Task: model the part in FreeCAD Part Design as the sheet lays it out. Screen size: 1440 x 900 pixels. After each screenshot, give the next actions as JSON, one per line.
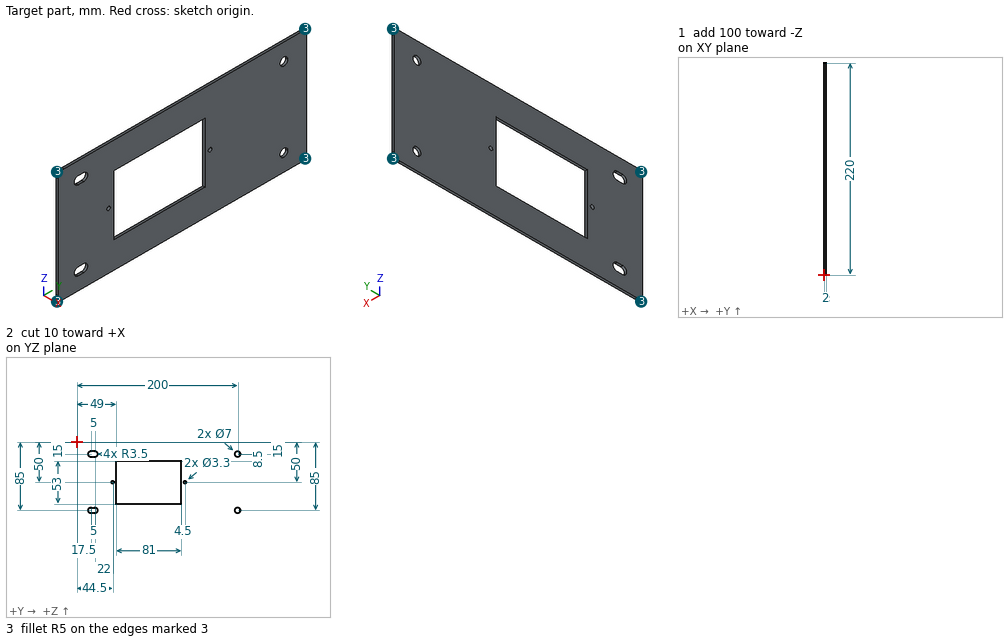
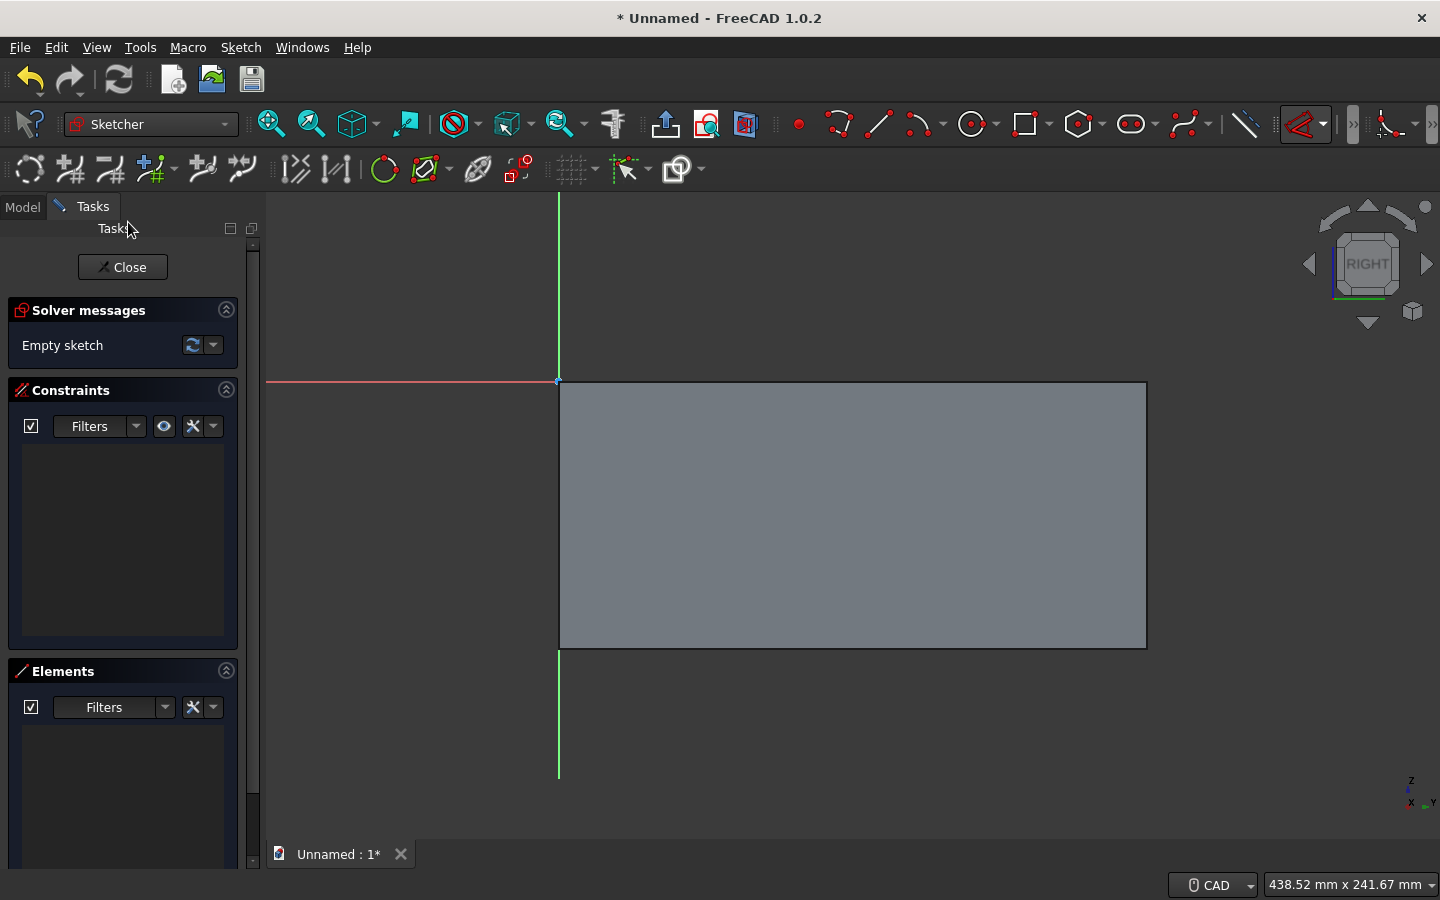
{"action": "left_click", "coordinate": [746, 124]}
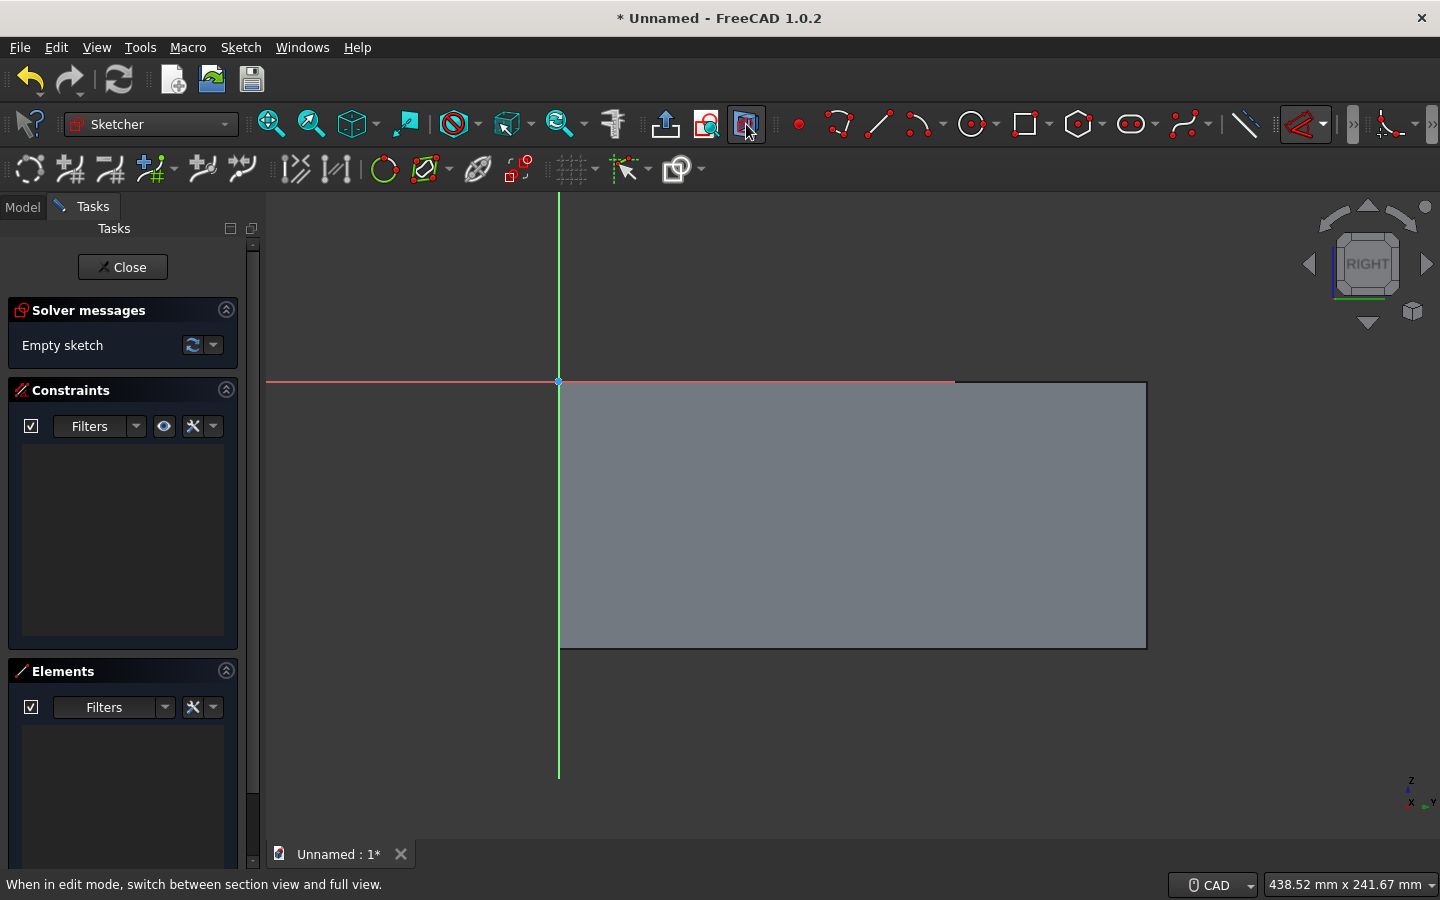
{"action": "left_click", "coordinate": [1026, 124]}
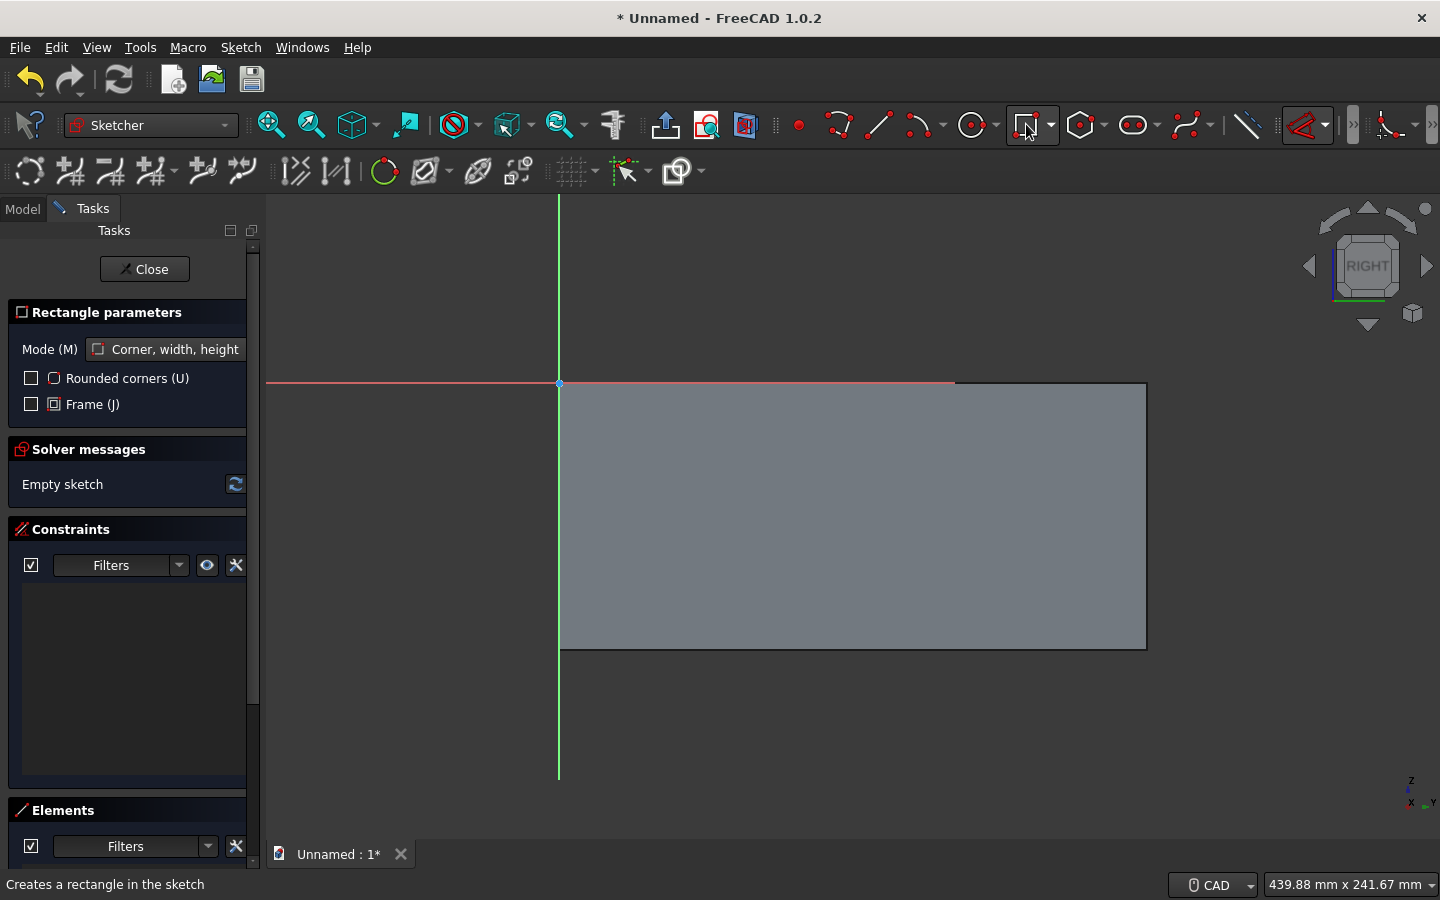
{"action": "left_click", "coordinate": [690, 446]}
{"action": "left_click", "coordinate": [906, 587]}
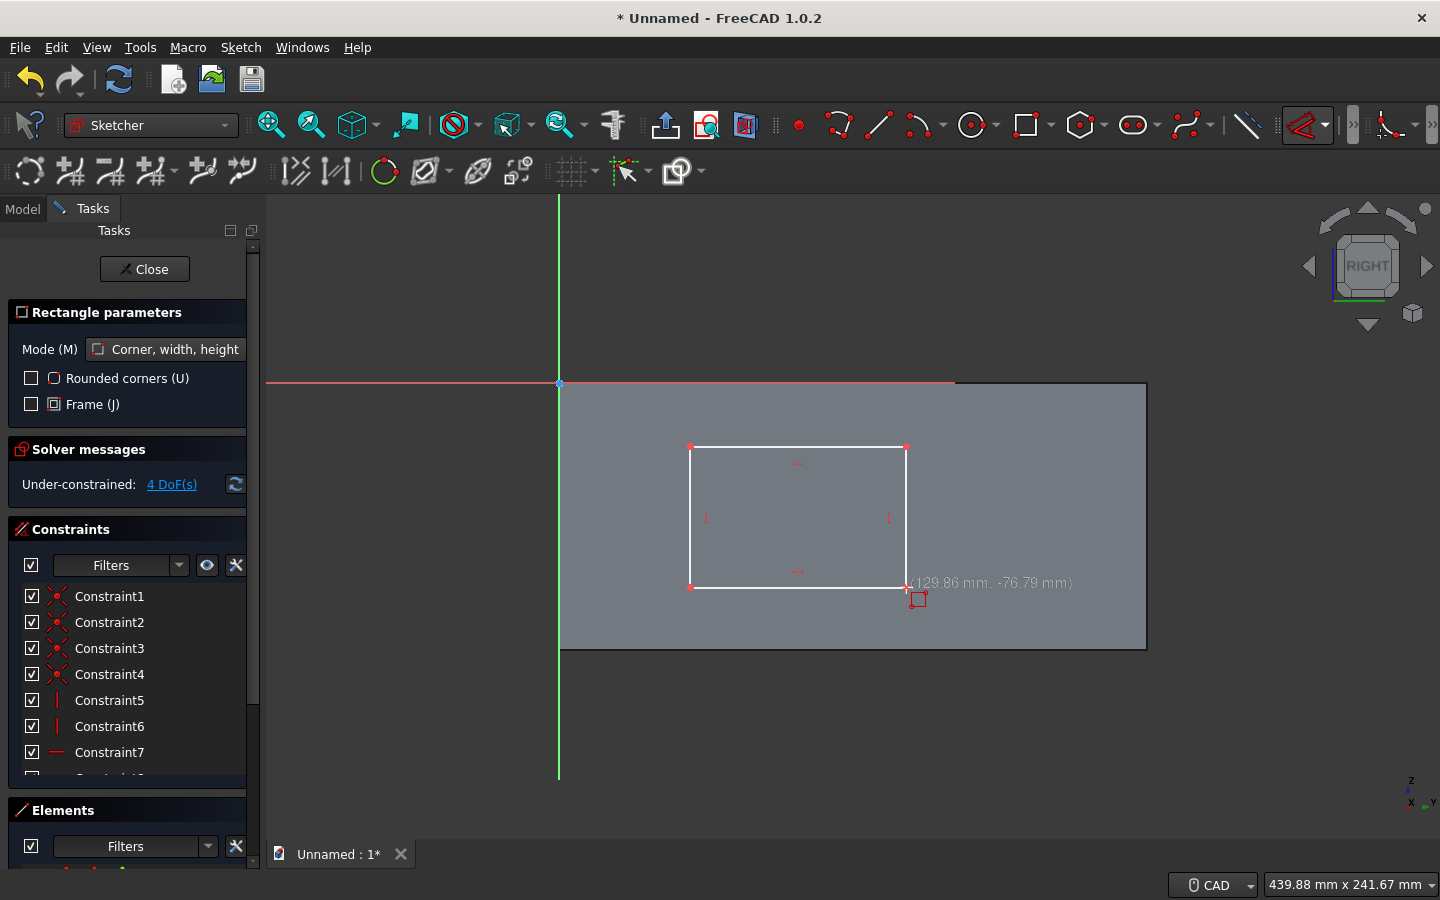
{"action": "left_click", "coordinate": [1134, 126]}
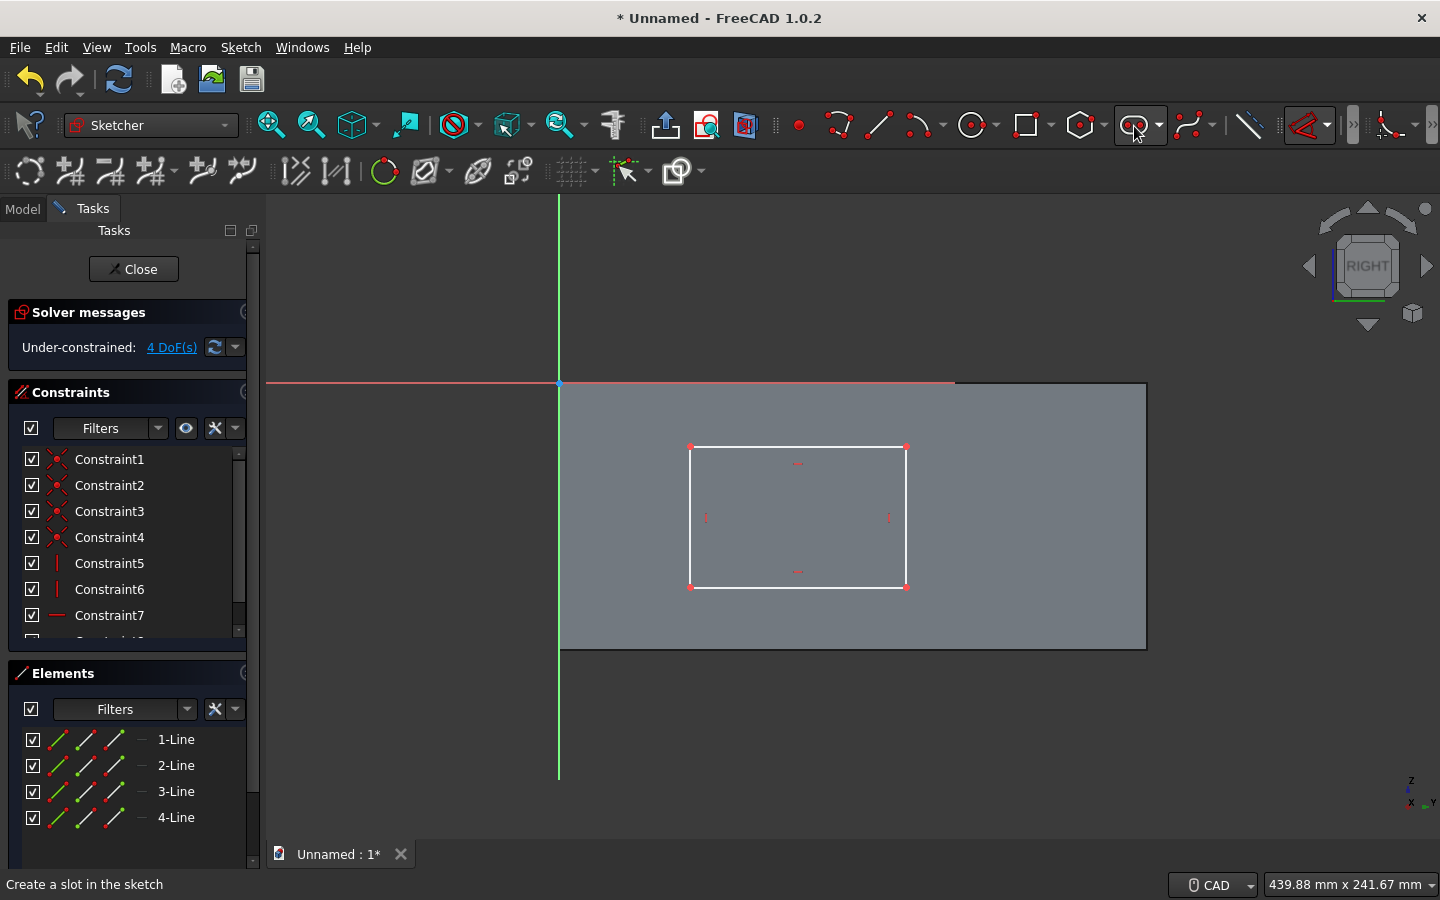
{"action": "scroll", "coordinate": [606, 423], "scroll_direction": "up", "scroll_amount": 5}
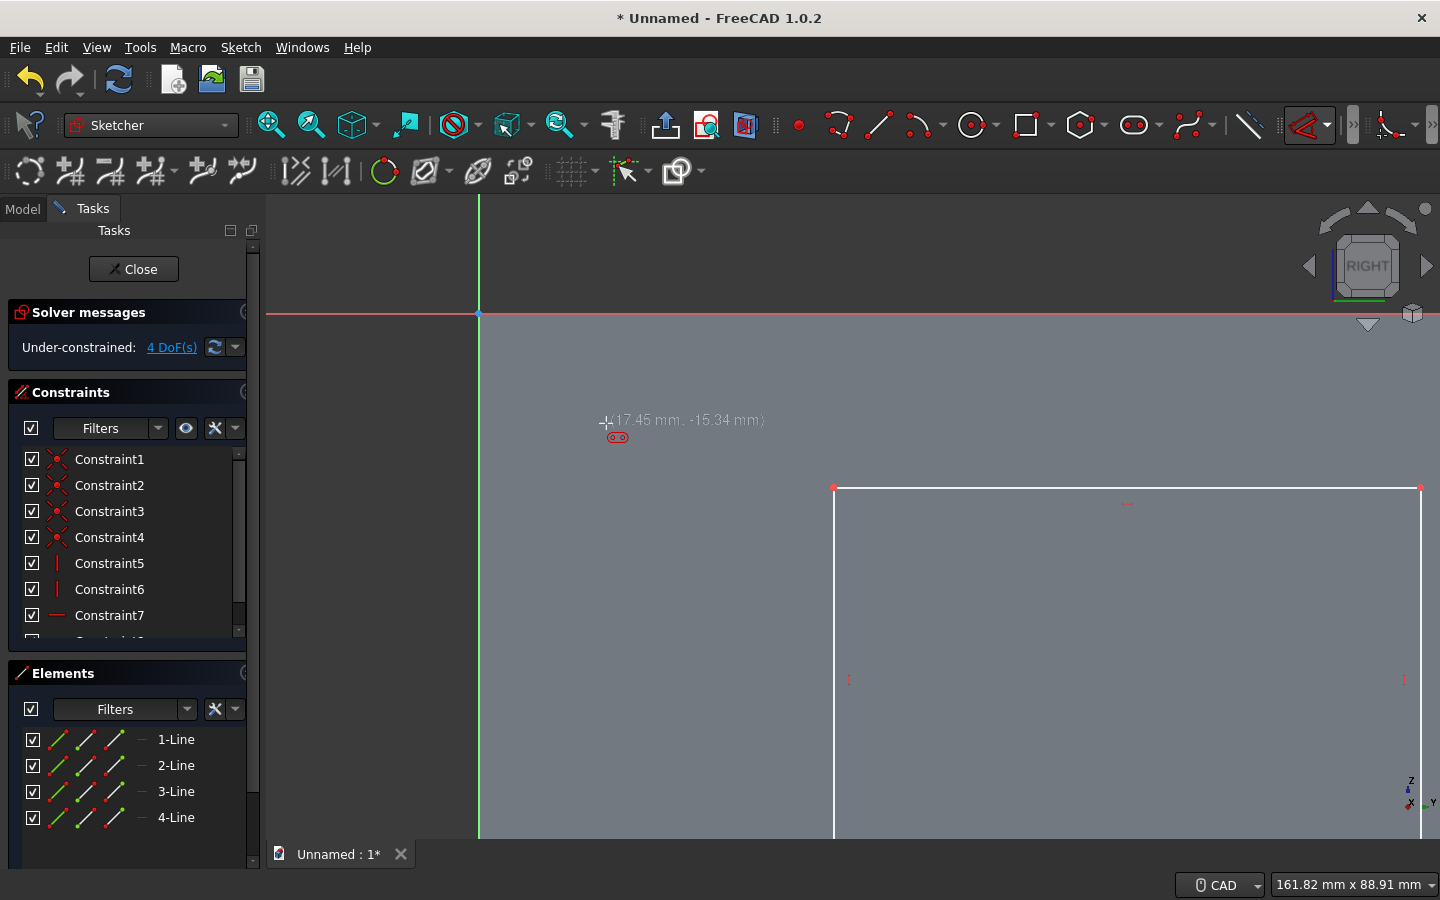
{"action": "left_click", "coordinate": [606, 423]}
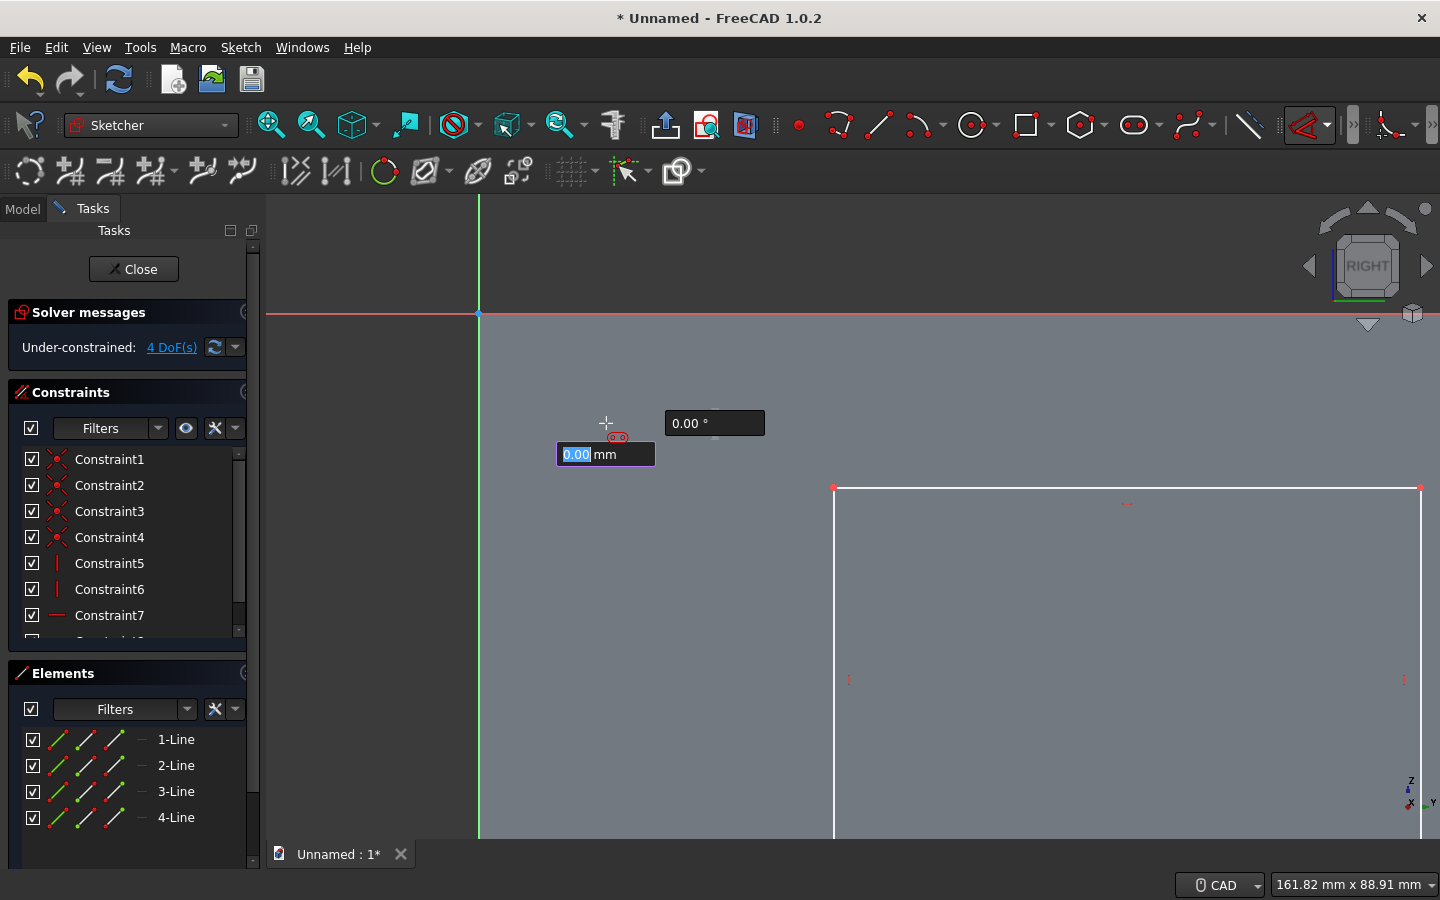
{"action": "left_click", "coordinate": [642, 423]}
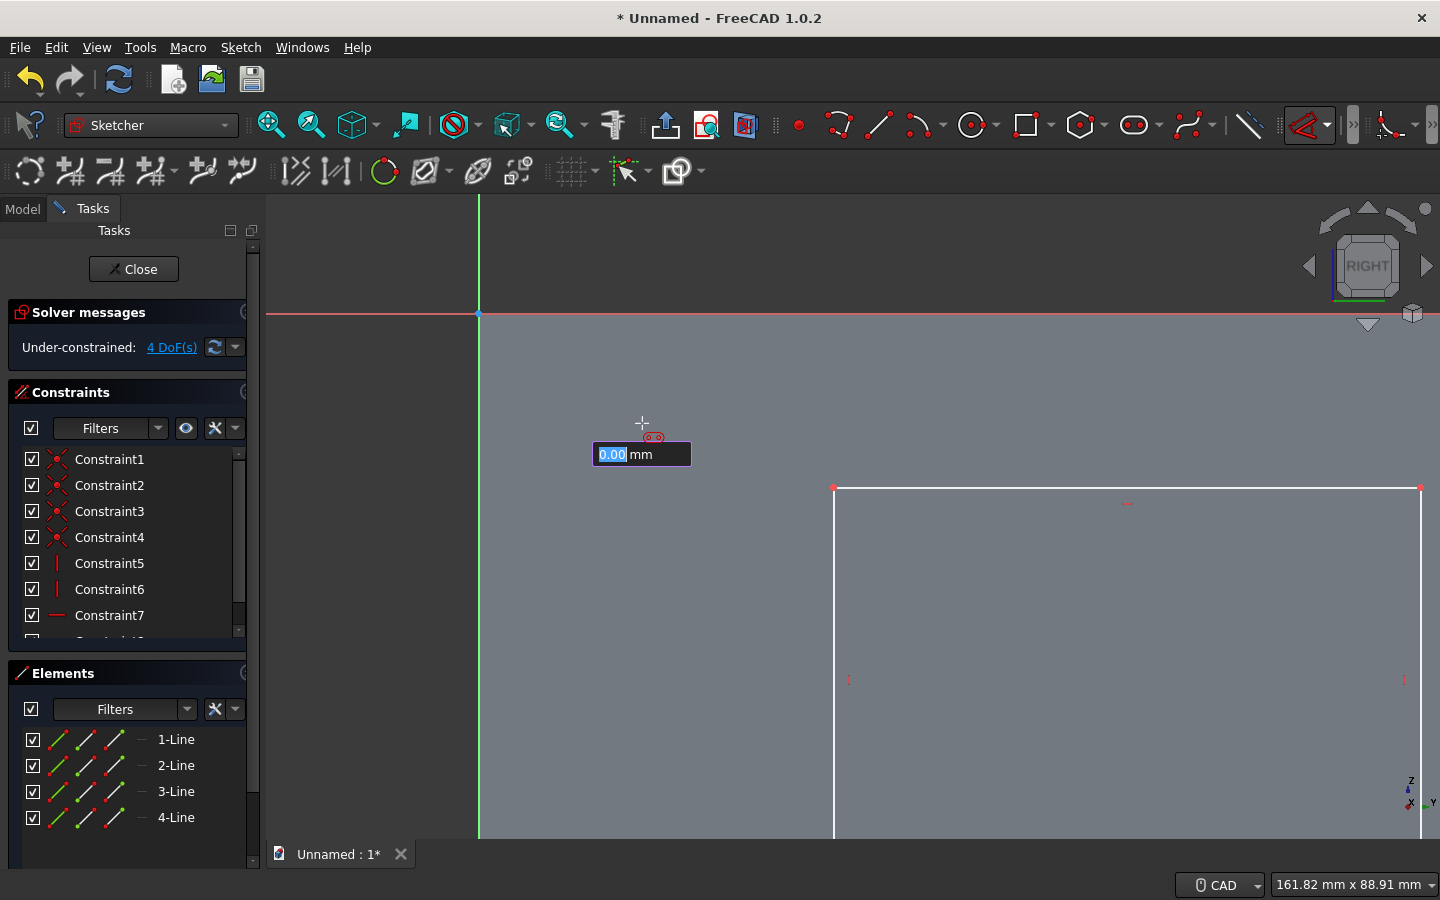
{"action": "left_click", "coordinate": [624, 397]}